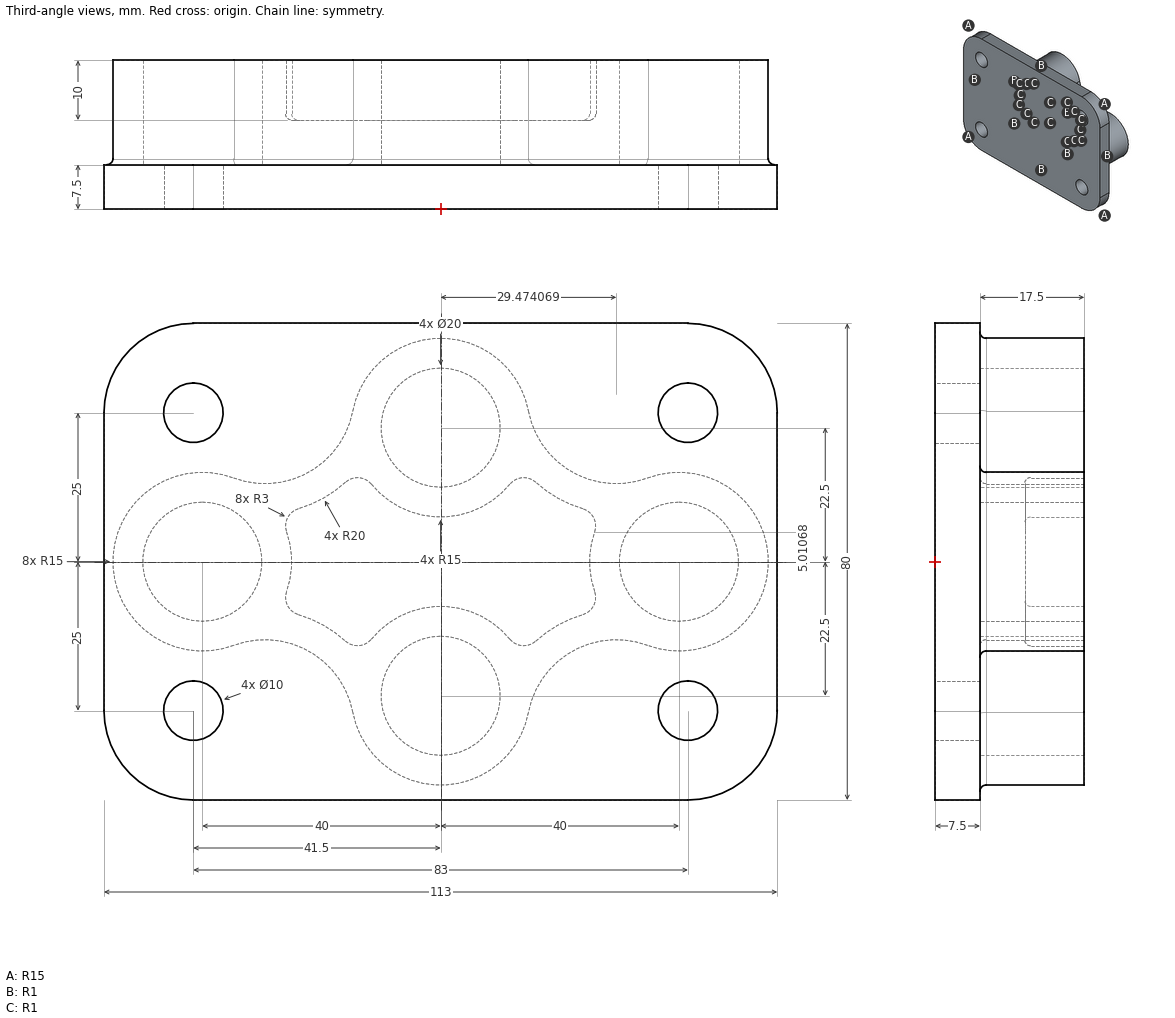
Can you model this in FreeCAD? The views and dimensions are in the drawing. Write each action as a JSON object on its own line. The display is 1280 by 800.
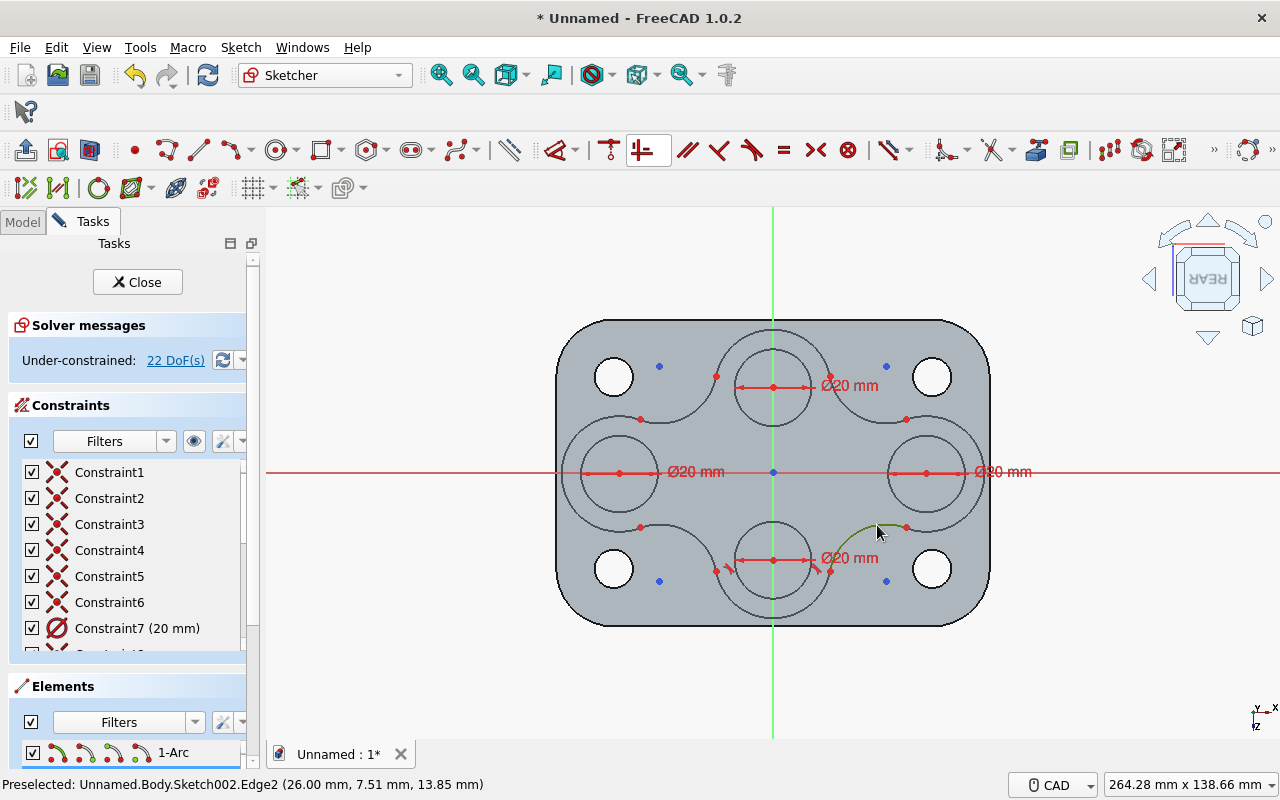
{"action": "left_click", "coordinate": [968, 514]}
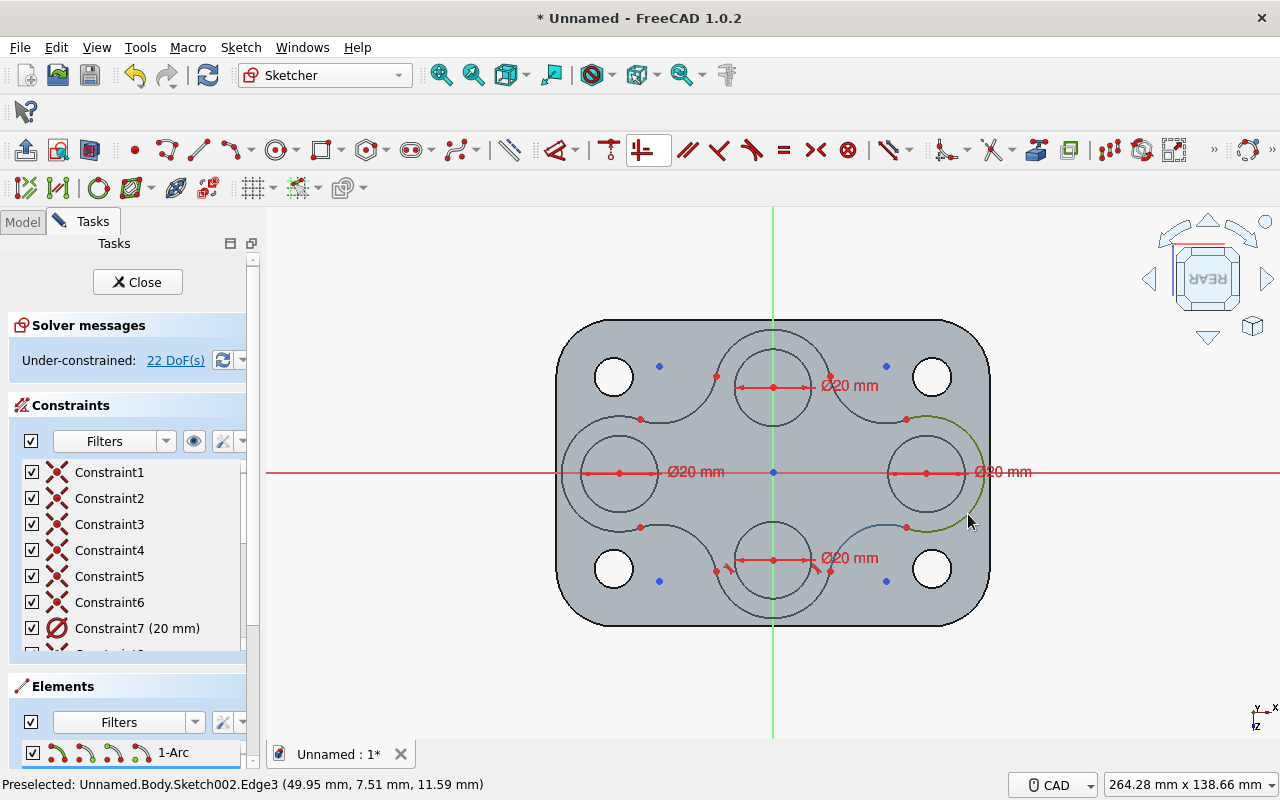
{"action": "left_click", "coordinate": [752, 150]}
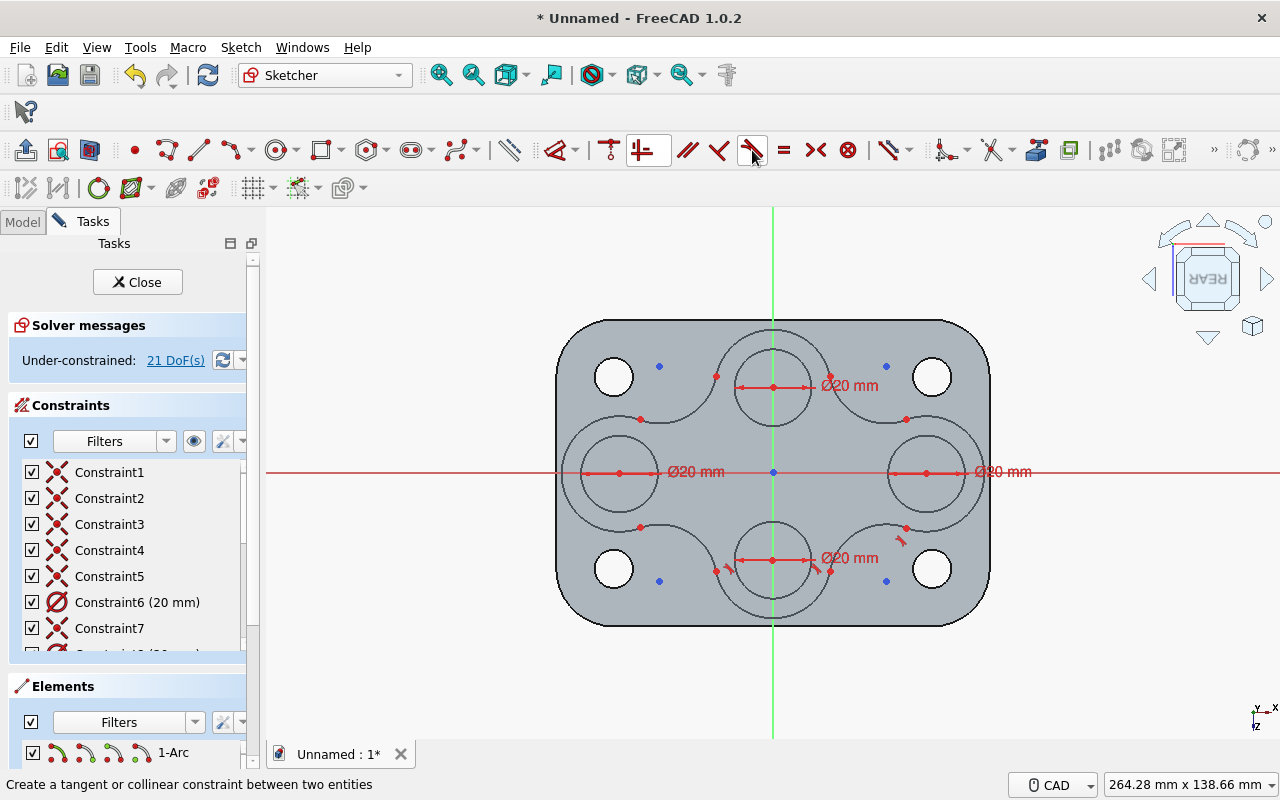
{"action": "left_click", "coordinate": [968, 514]}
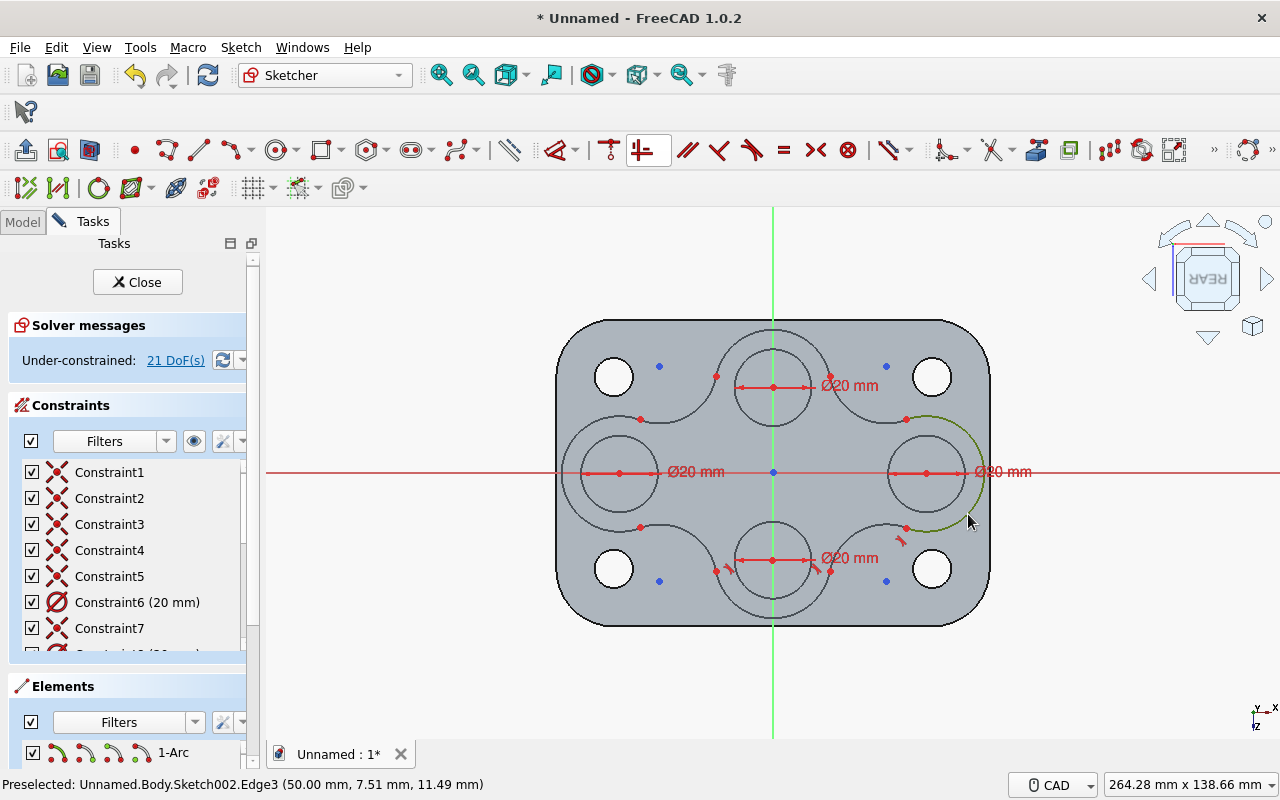
{"action": "left_click", "coordinate": [843, 404]}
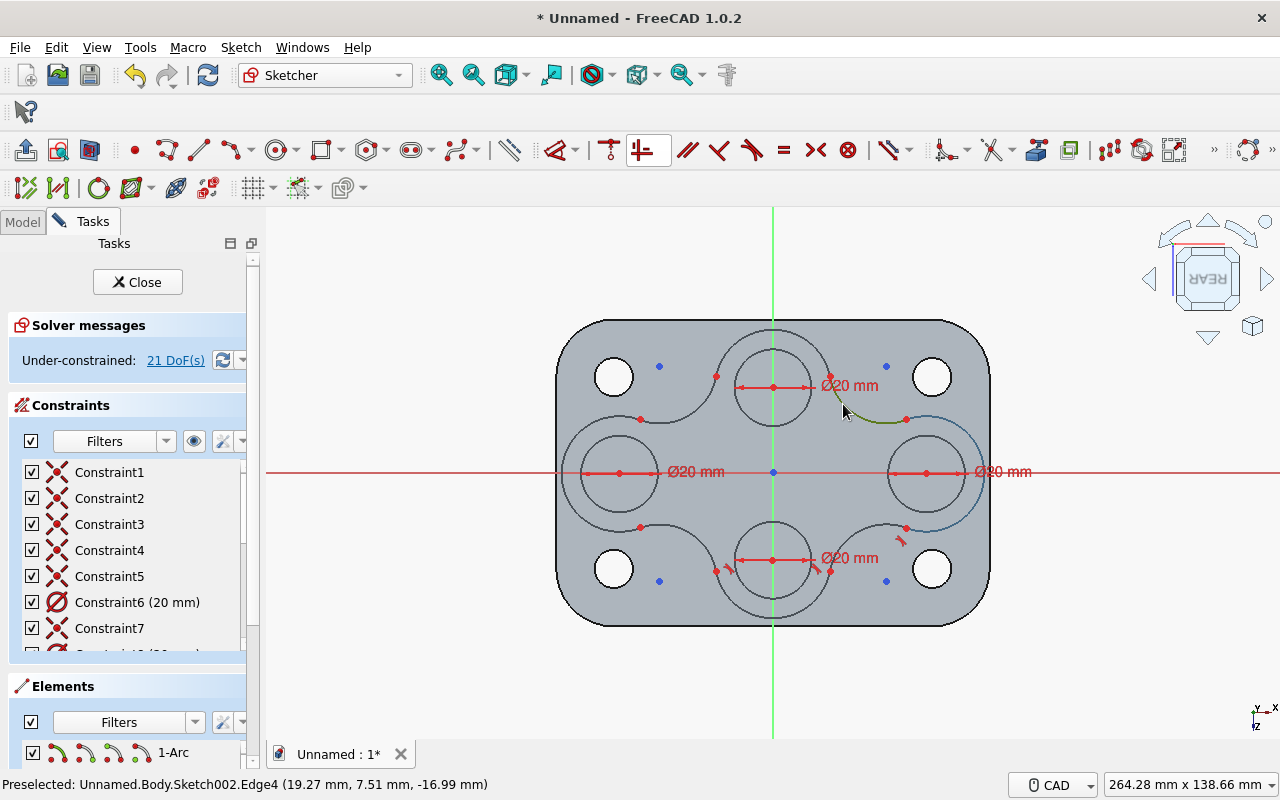
{"action": "key", "text": "t"}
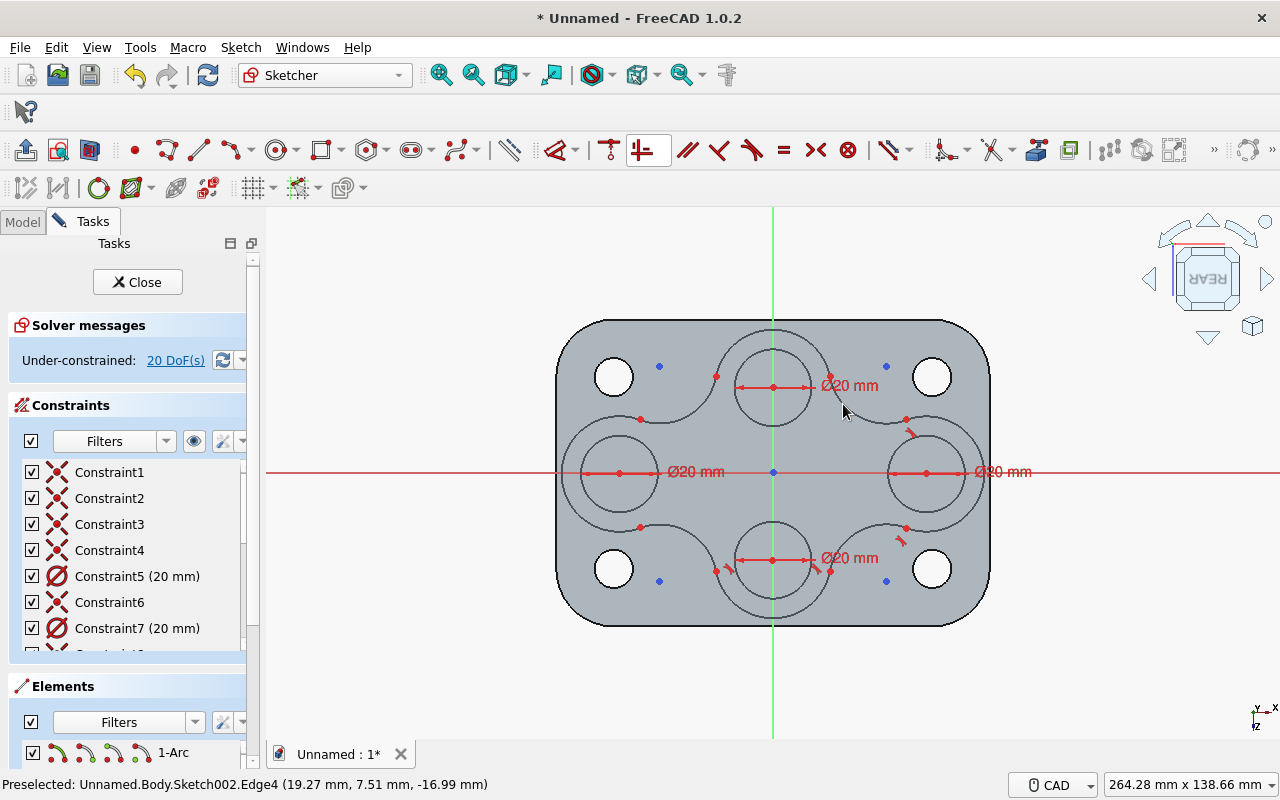
{"action": "left_click", "coordinate": [843, 404]}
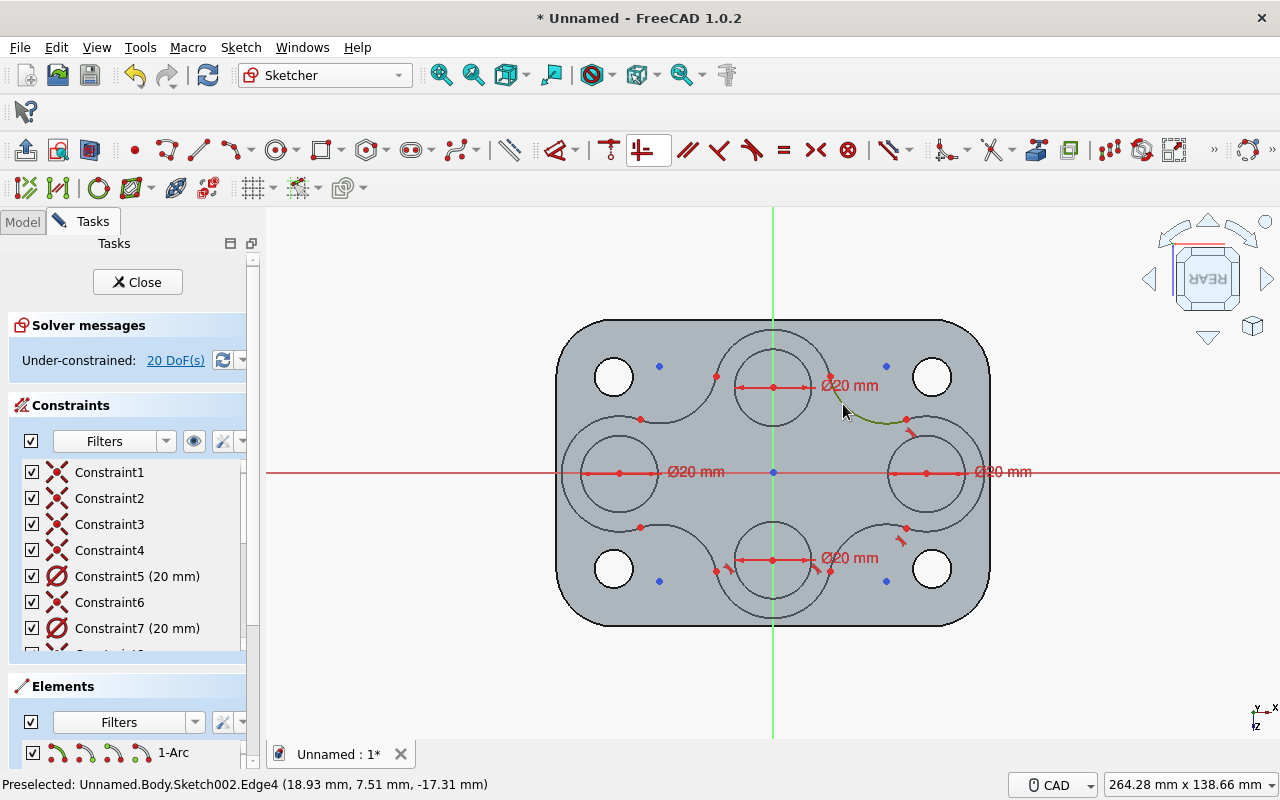
{"action": "left_click", "coordinate": [804, 338]}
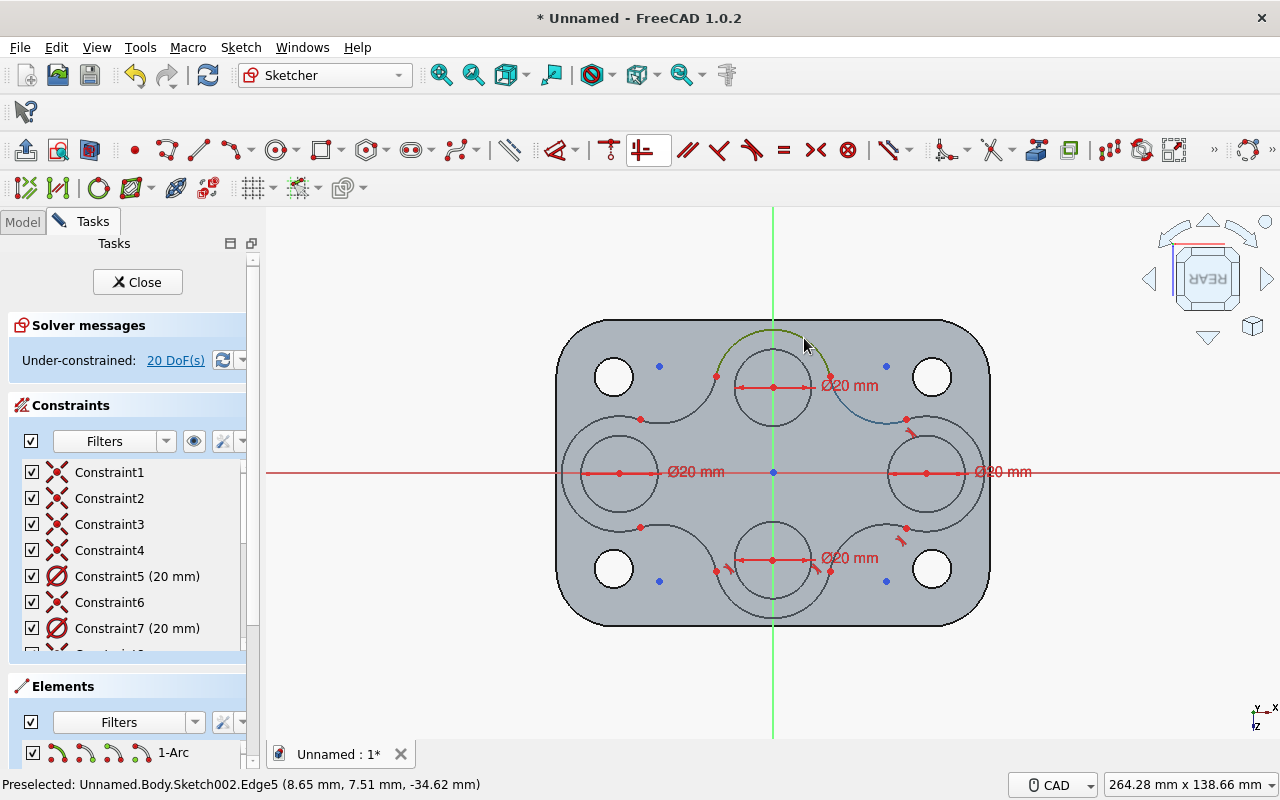
{"action": "key", "text": "t"}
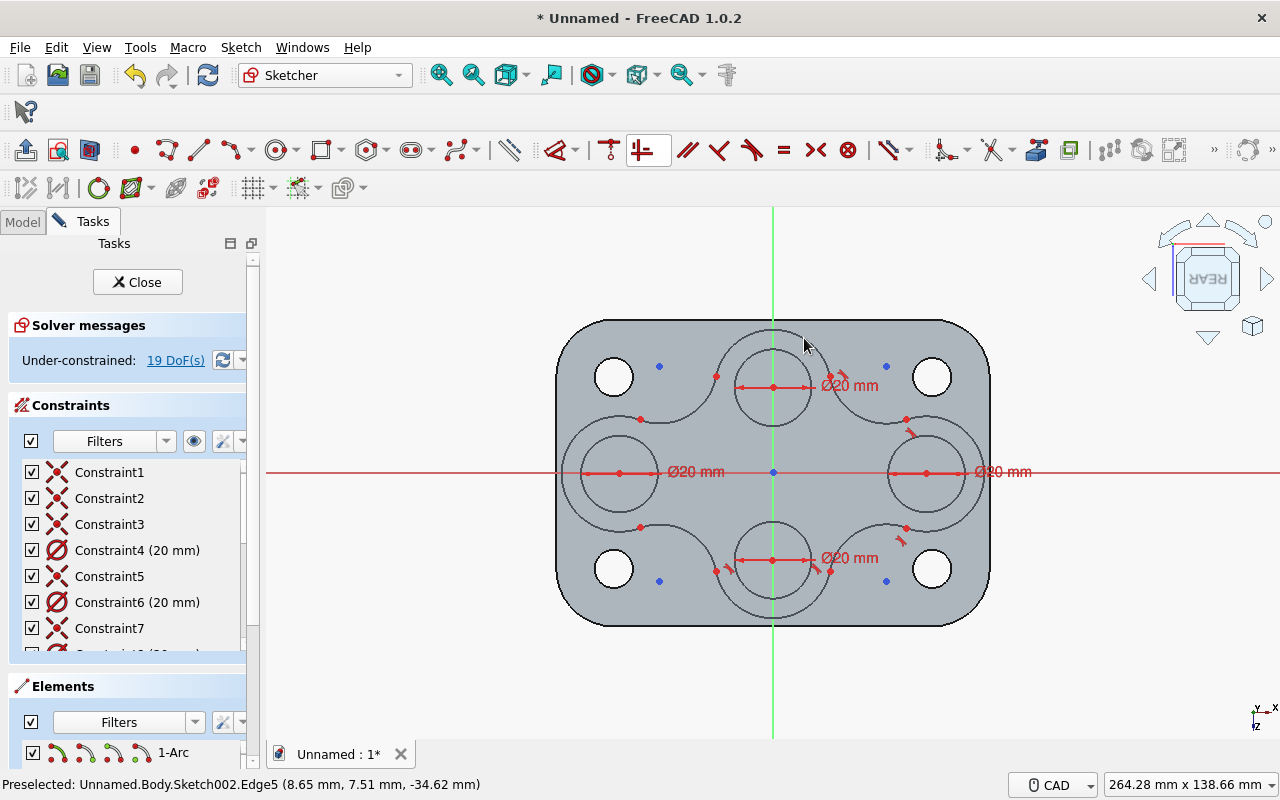
{"action": "left_click", "coordinate": [803, 338]}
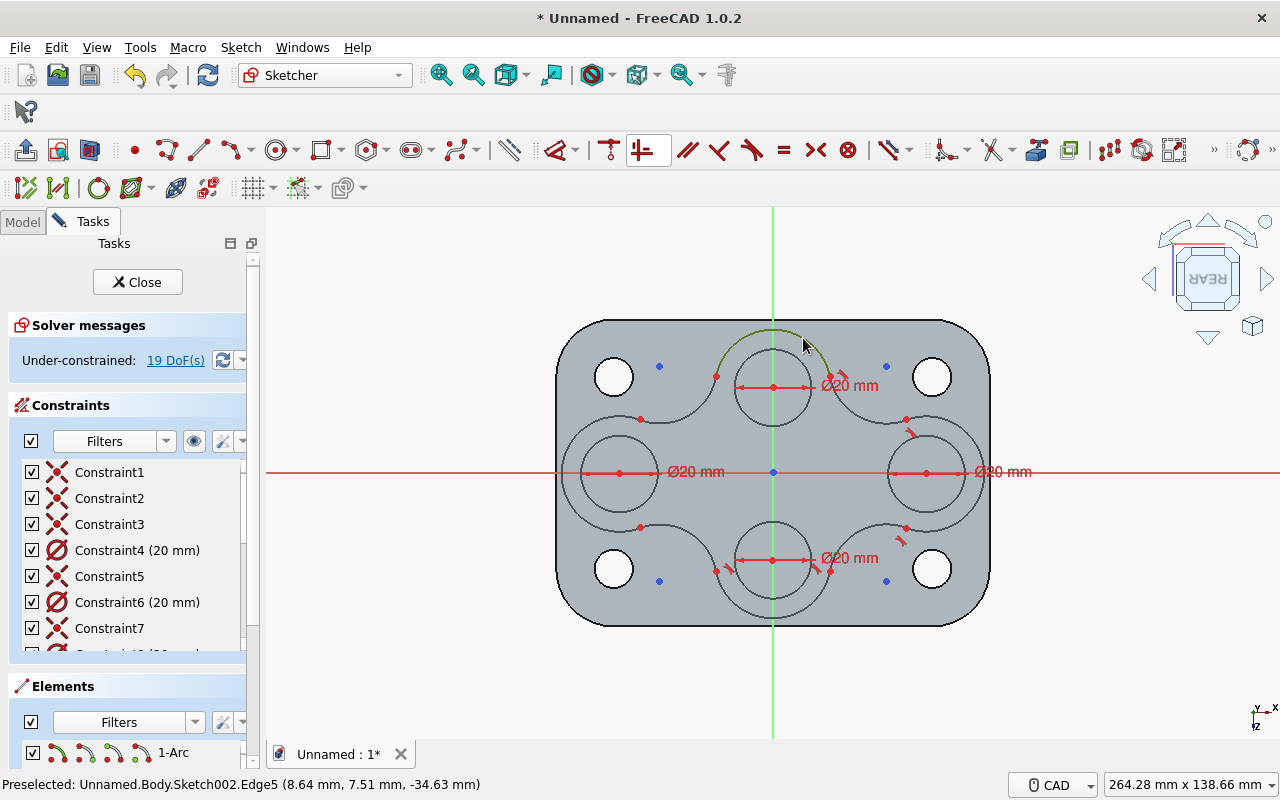
{"action": "left_click", "coordinate": [669, 423]}